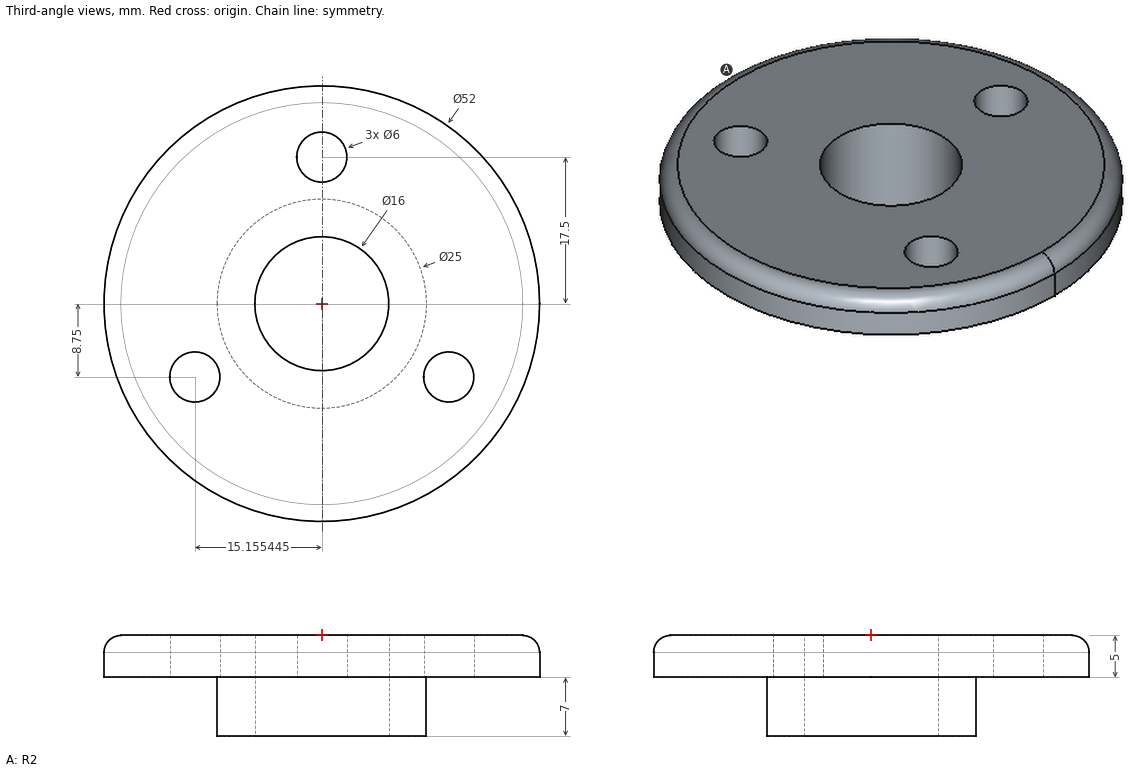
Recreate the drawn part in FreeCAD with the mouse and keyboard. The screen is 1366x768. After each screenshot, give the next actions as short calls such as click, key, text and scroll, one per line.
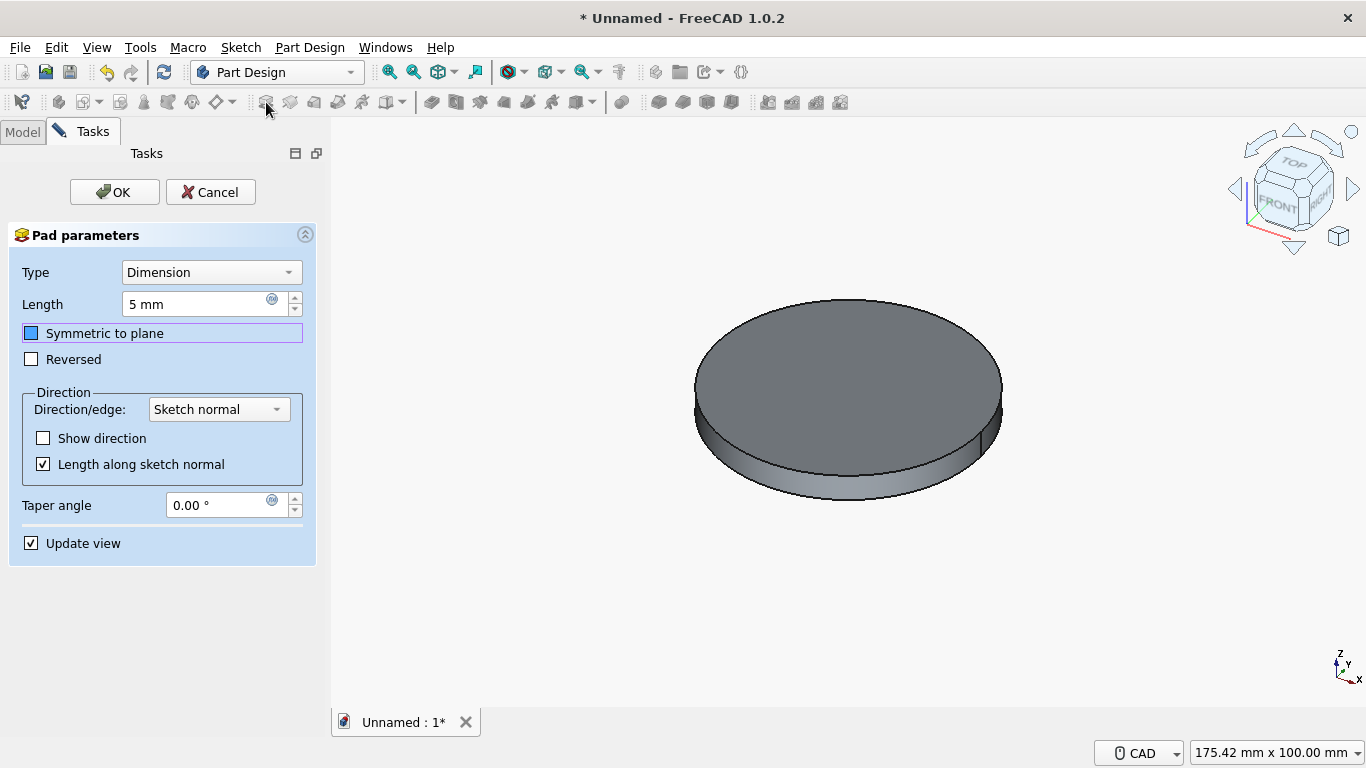
click(30, 359)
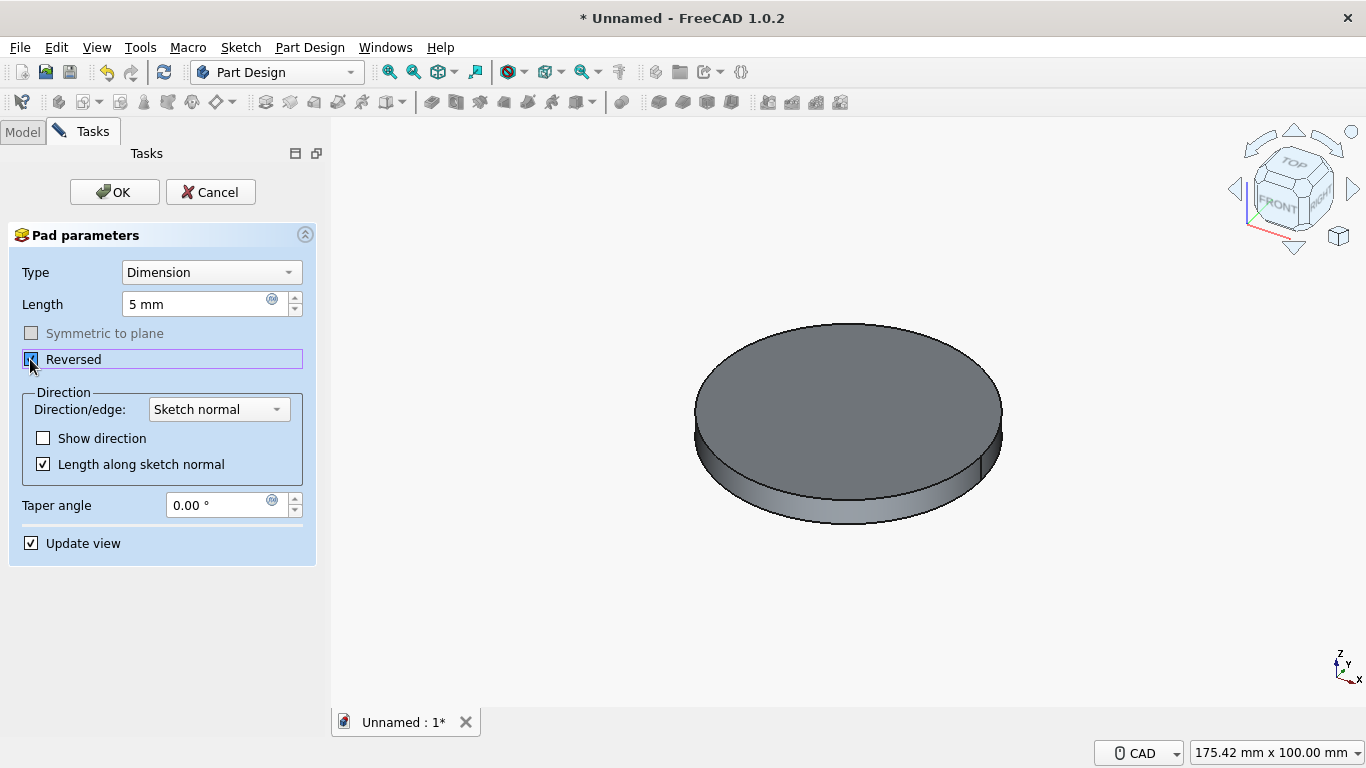
click(115, 192)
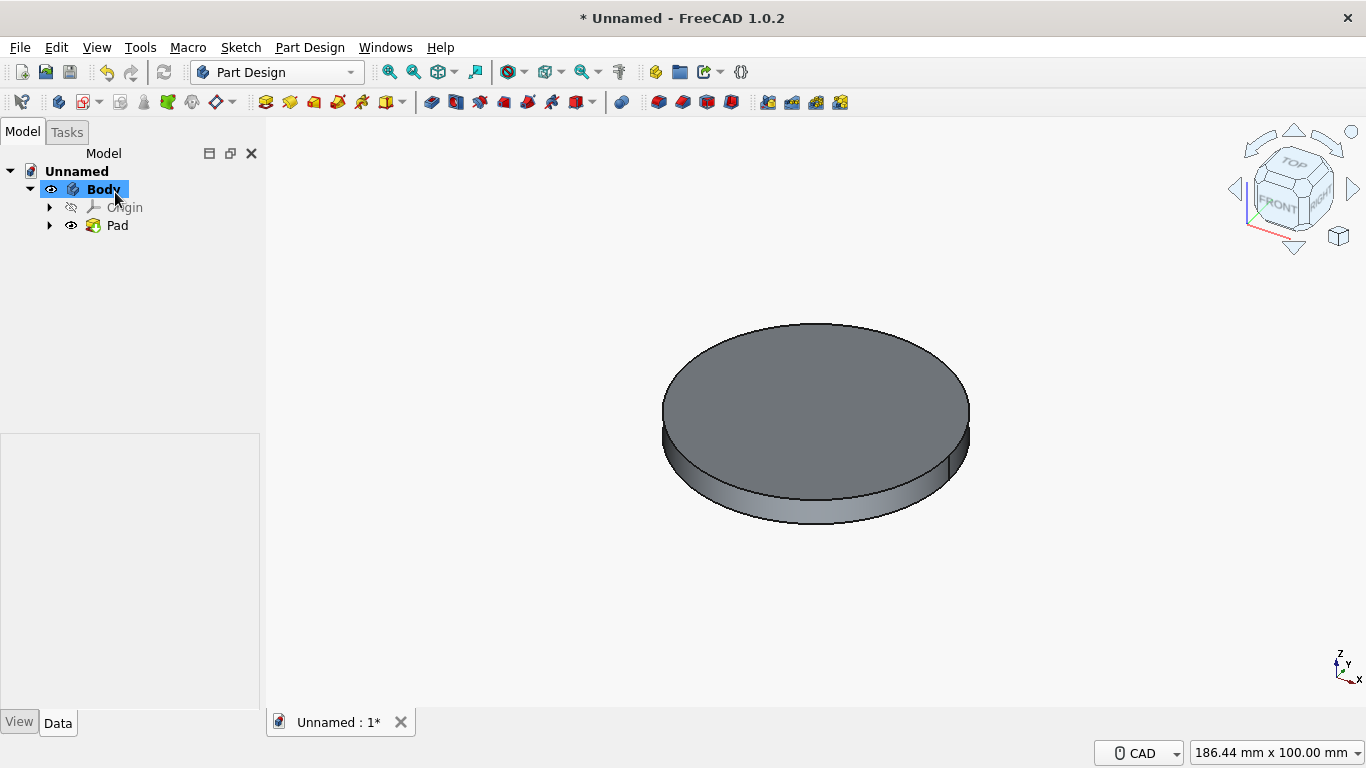
click(390, 72)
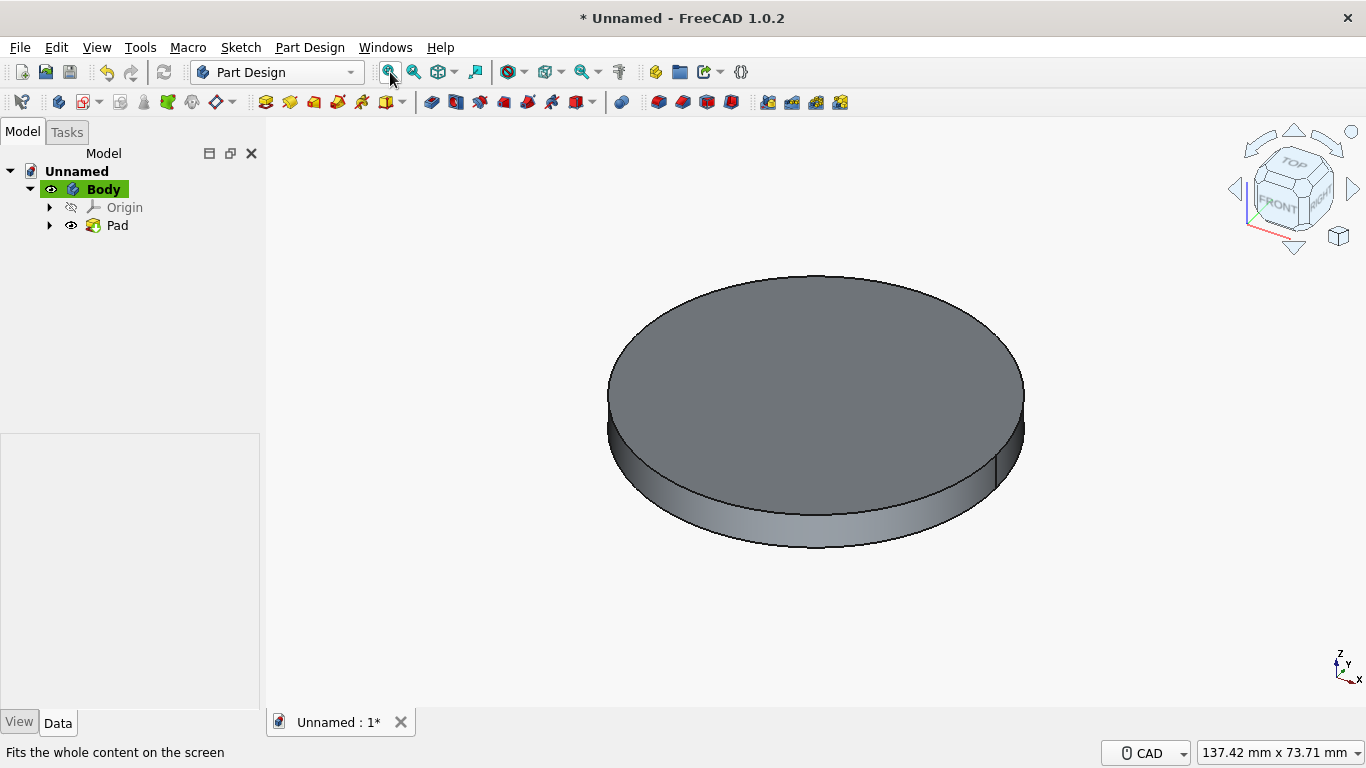
key(5)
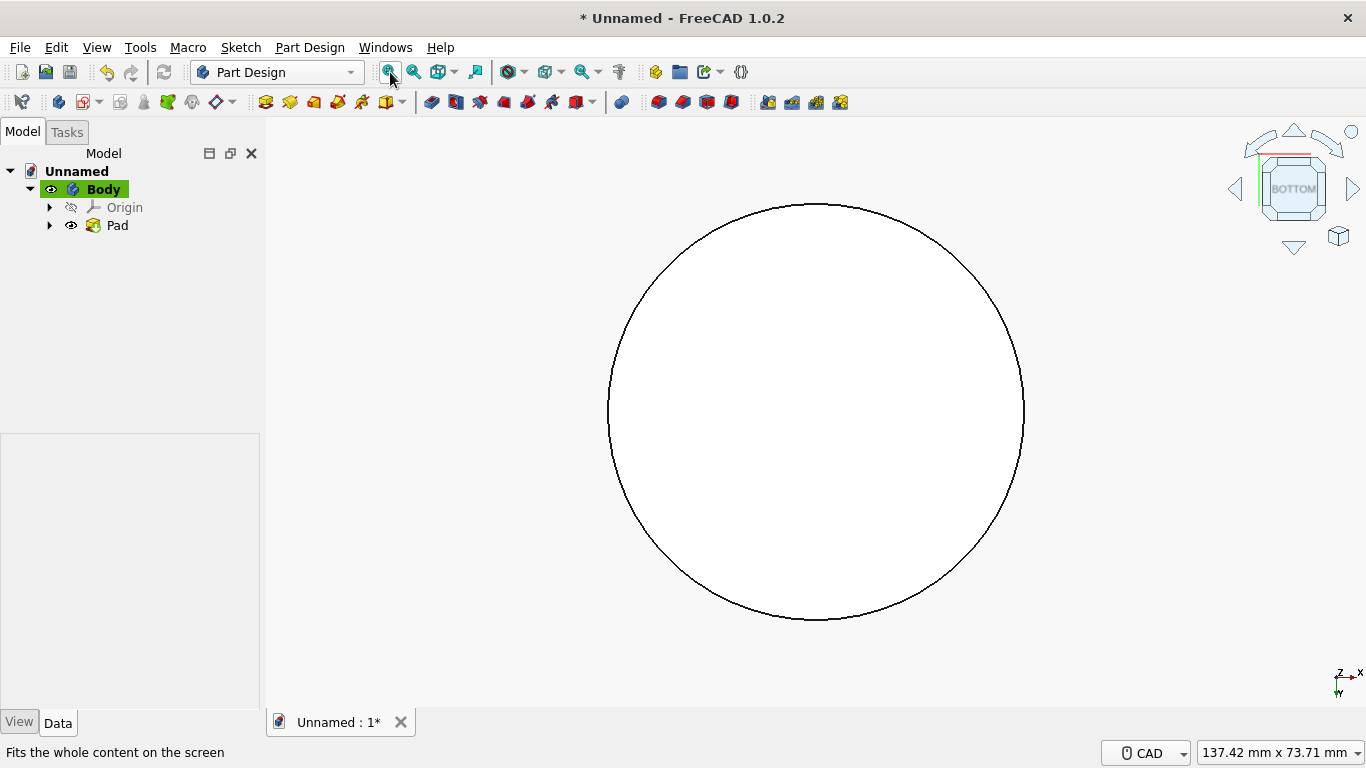
click(816, 411)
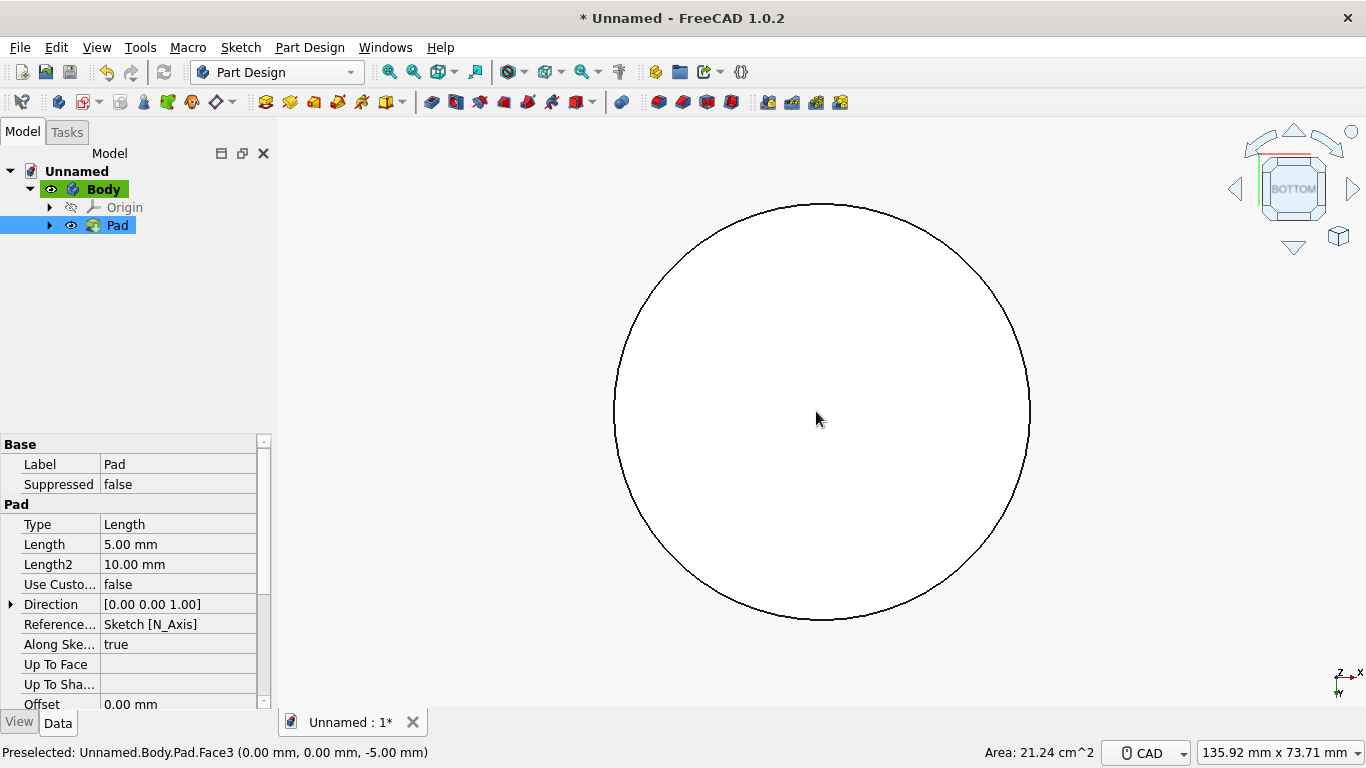
click(84, 102)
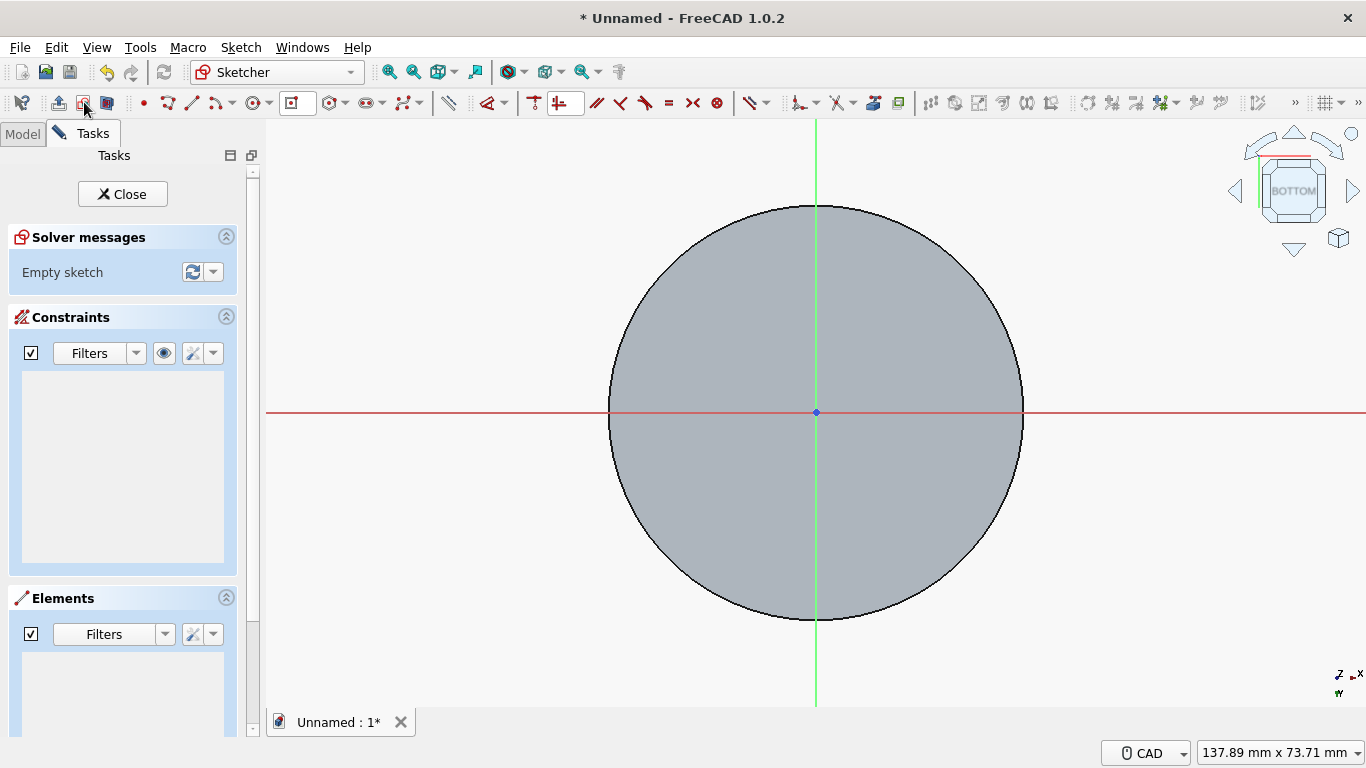
scroll(899, 413, up, 3)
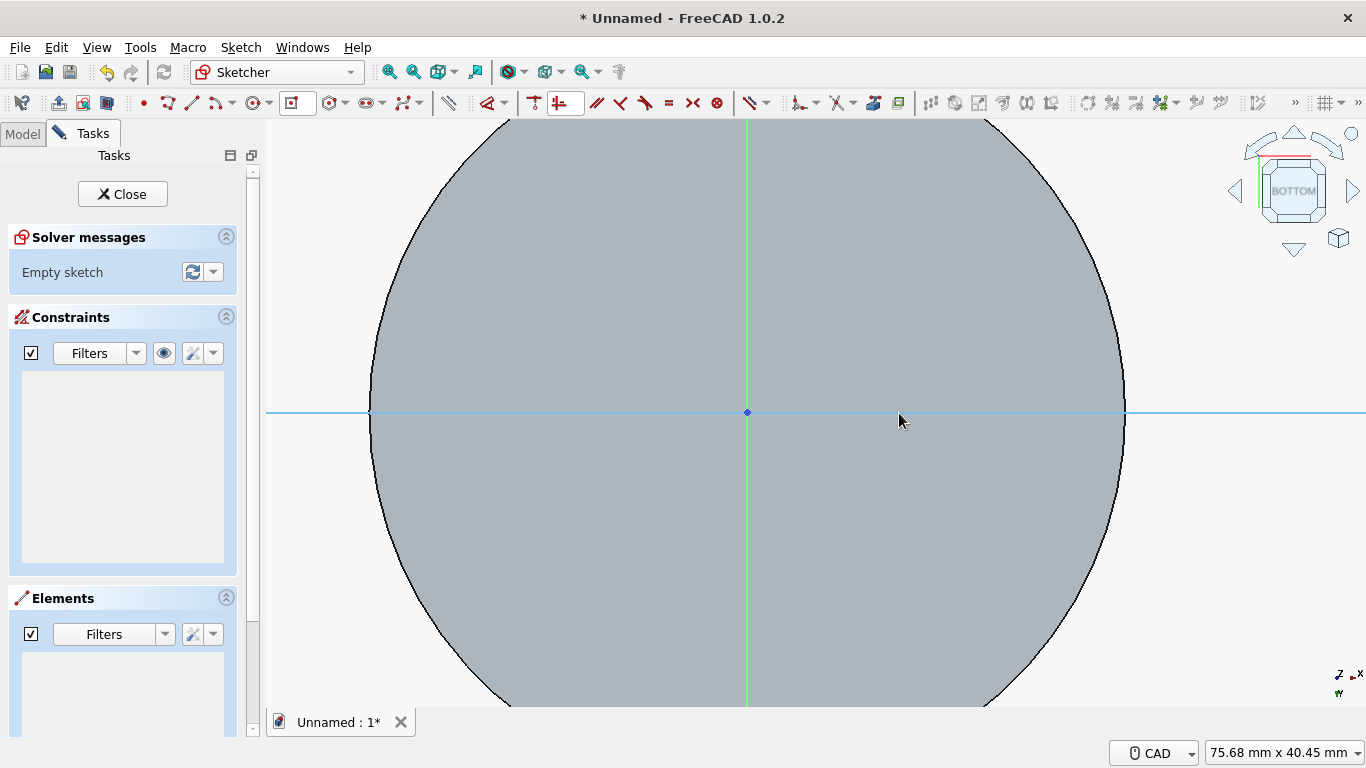
click(254, 104)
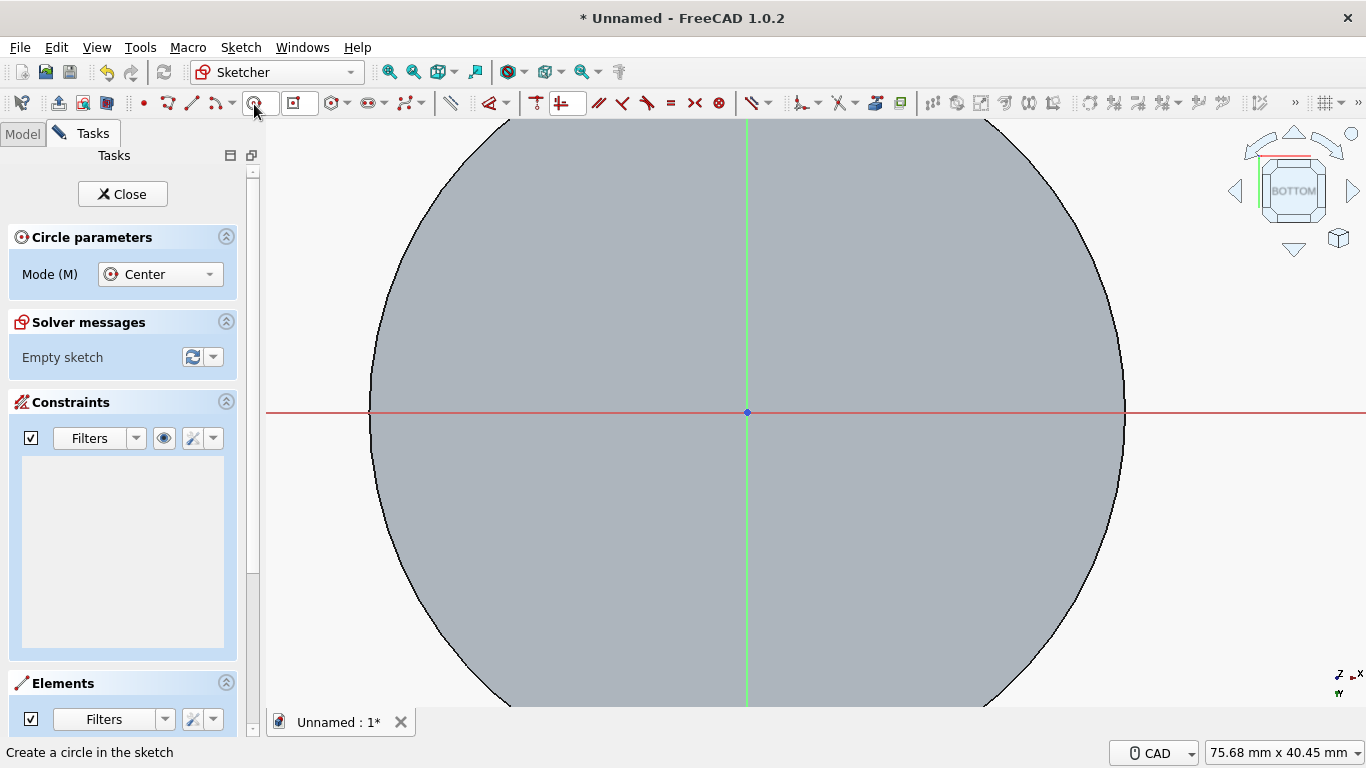
click(747, 413)
move(876, 284)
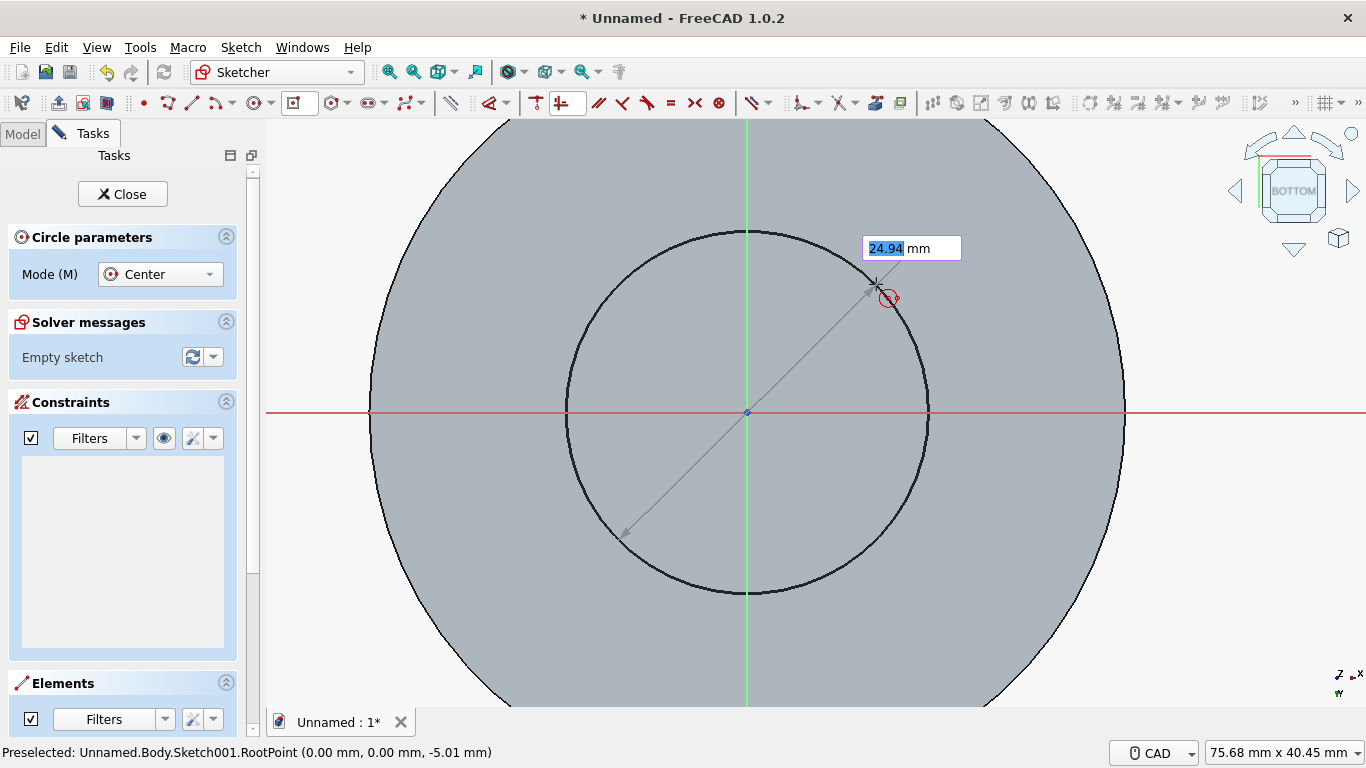
text(25)
key(Return)
key(Escape)